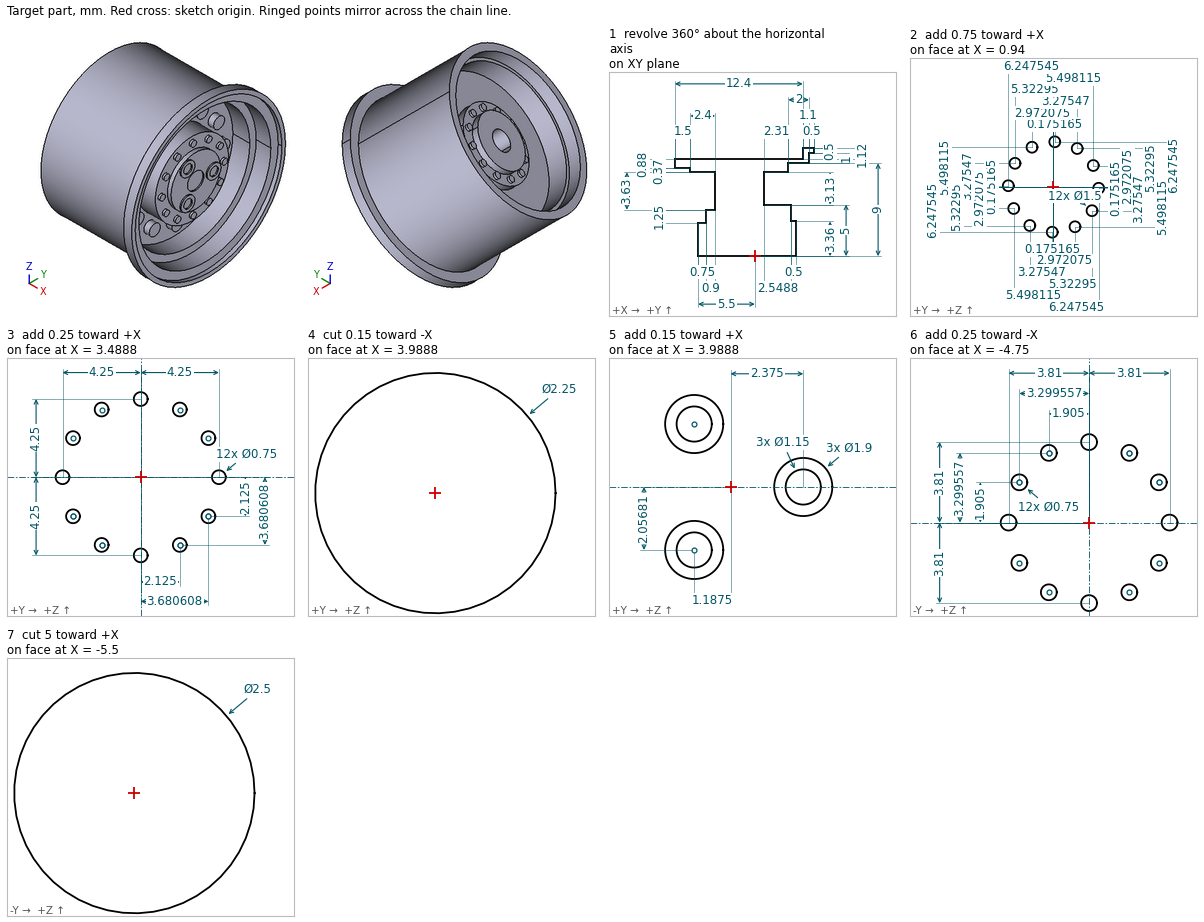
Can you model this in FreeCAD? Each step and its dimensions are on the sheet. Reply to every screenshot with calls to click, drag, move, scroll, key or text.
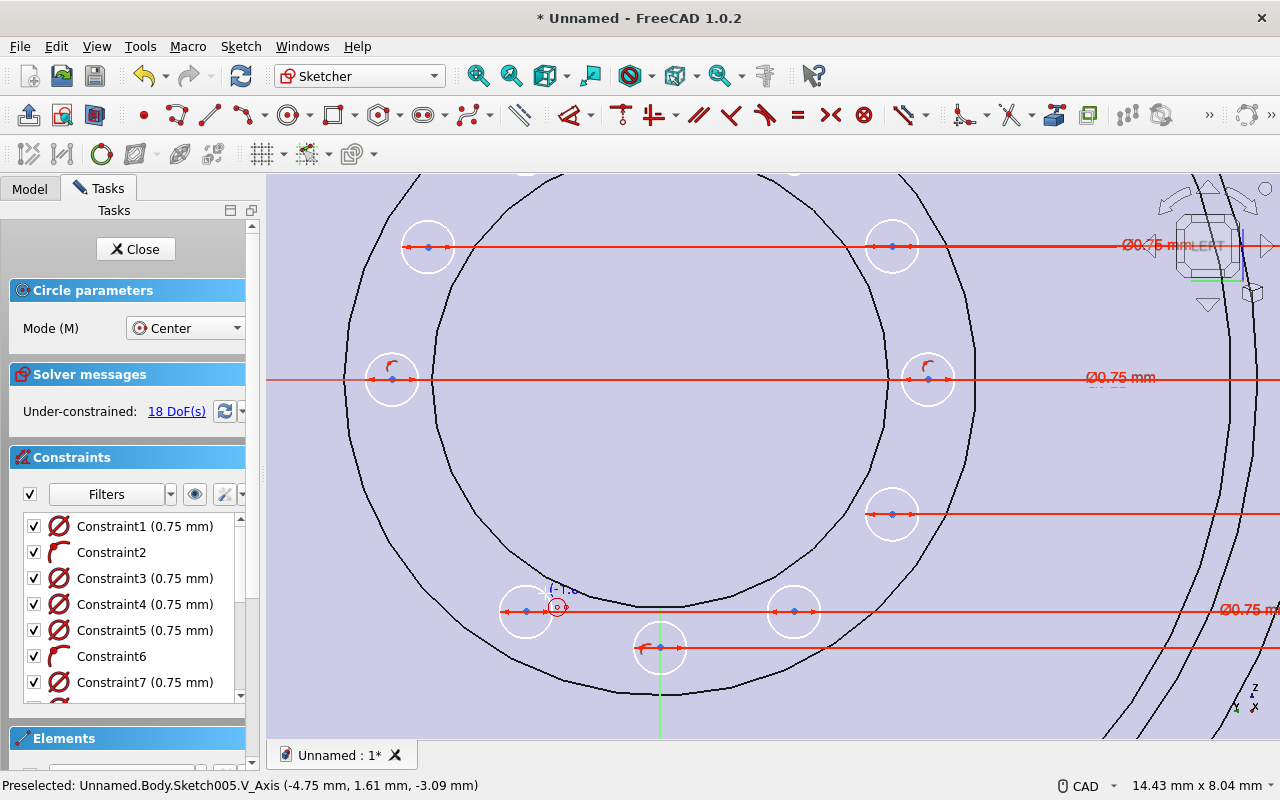
click(428, 513)
move(447, 495)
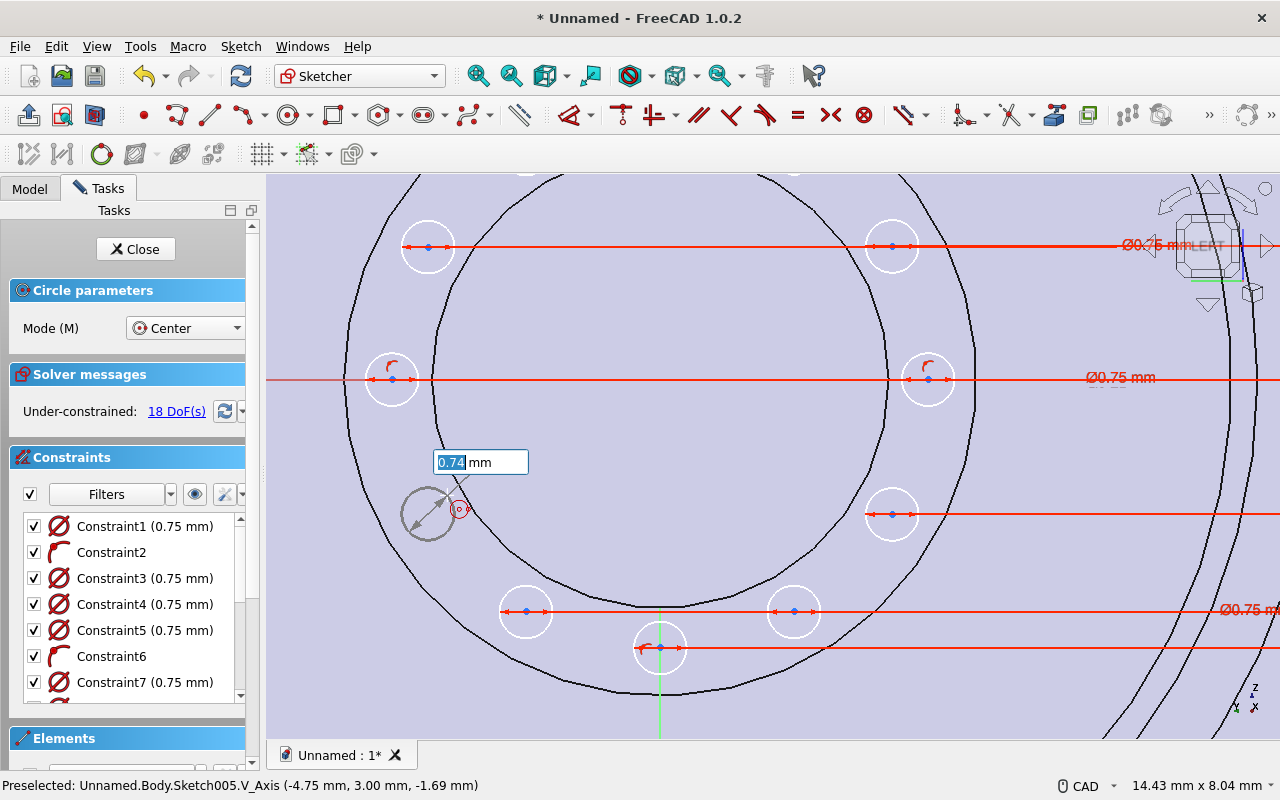
text(0.75)
key(Return)
key(Escape)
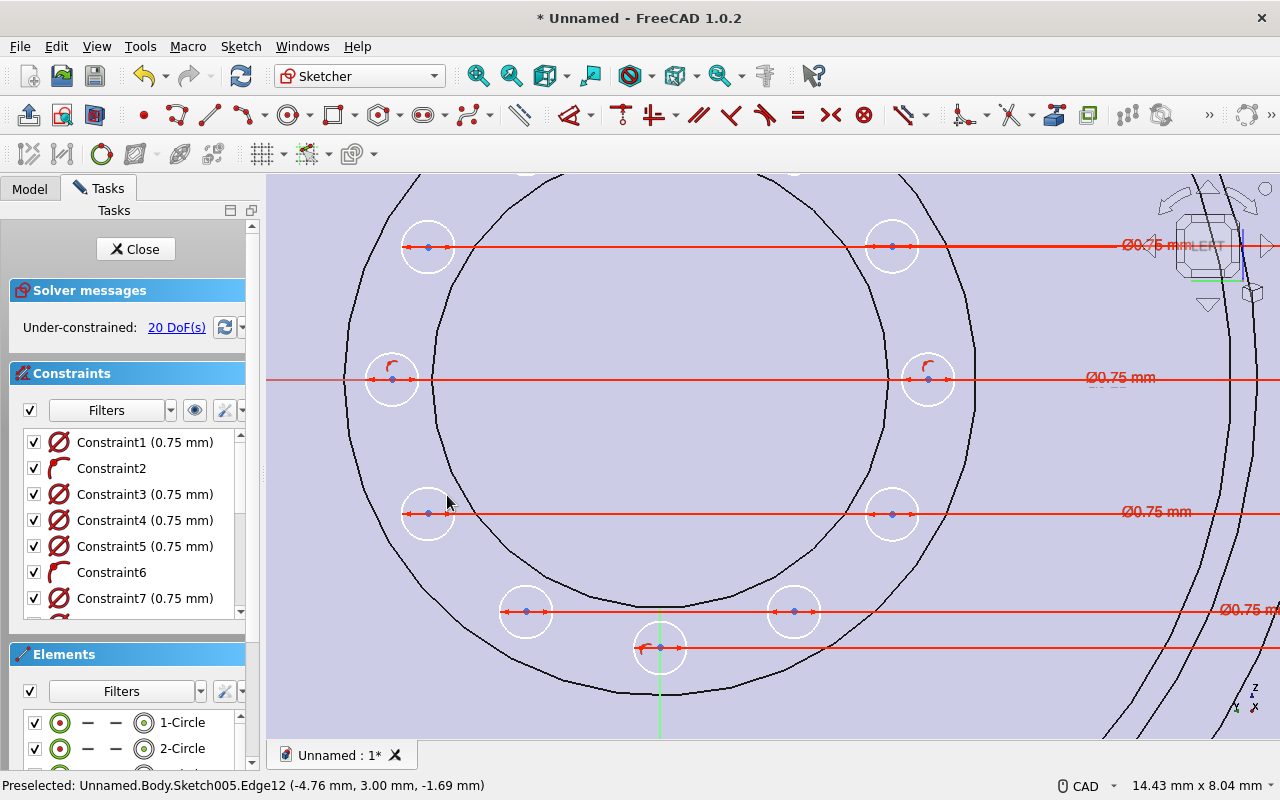
scroll(794, 613, down, 2)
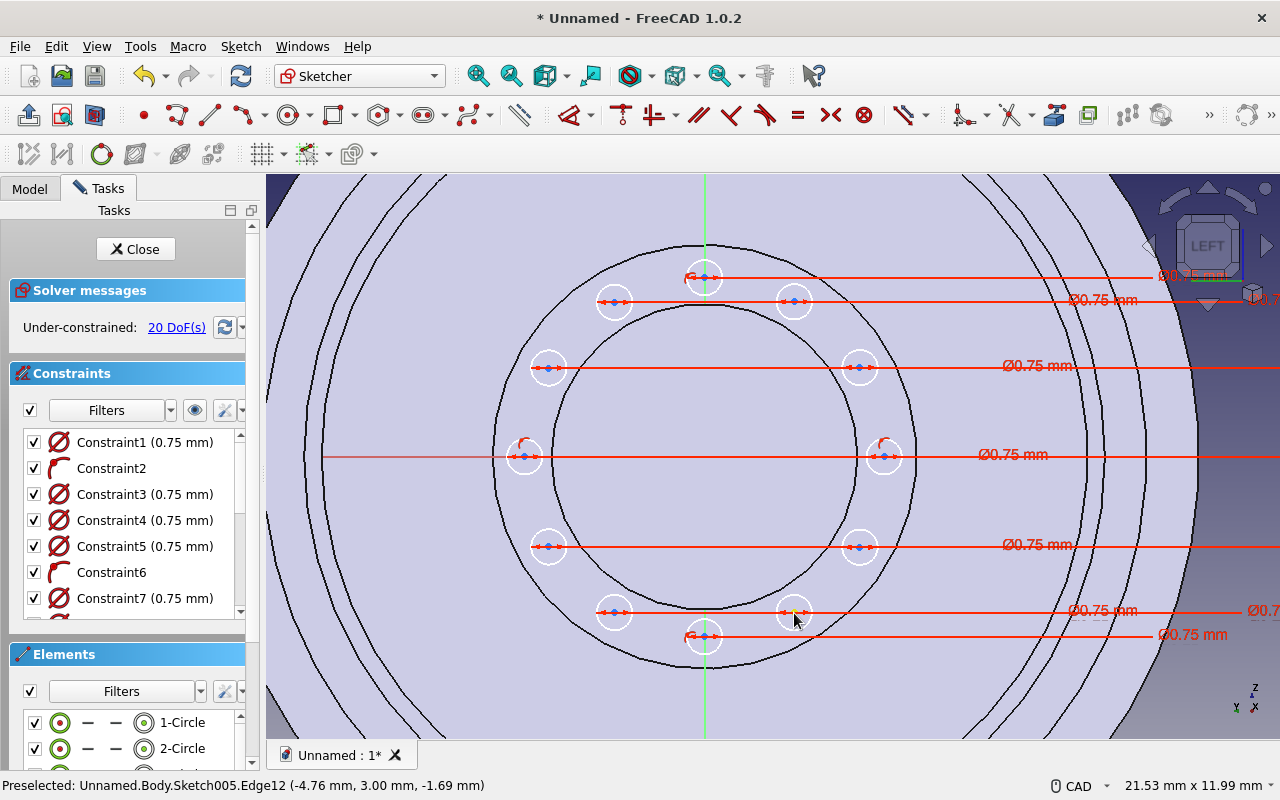
click(615, 302)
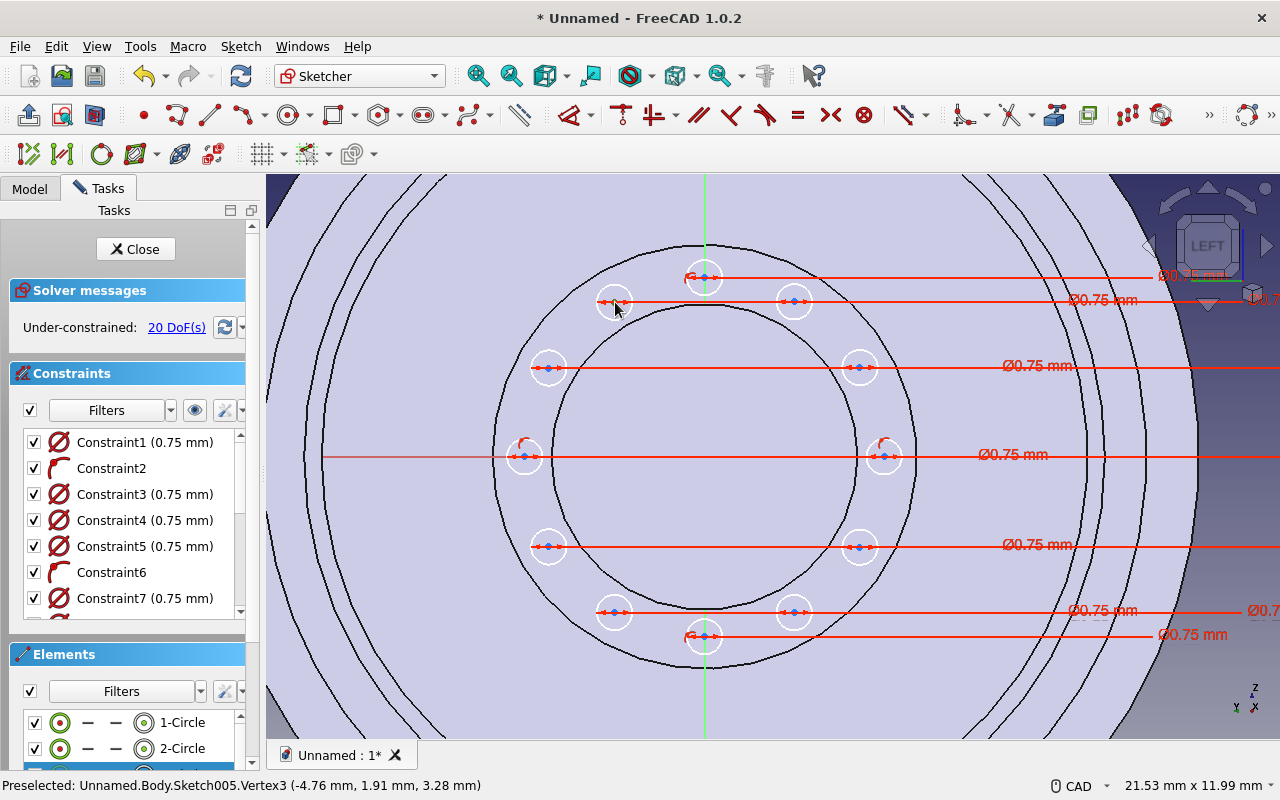
click(794, 302)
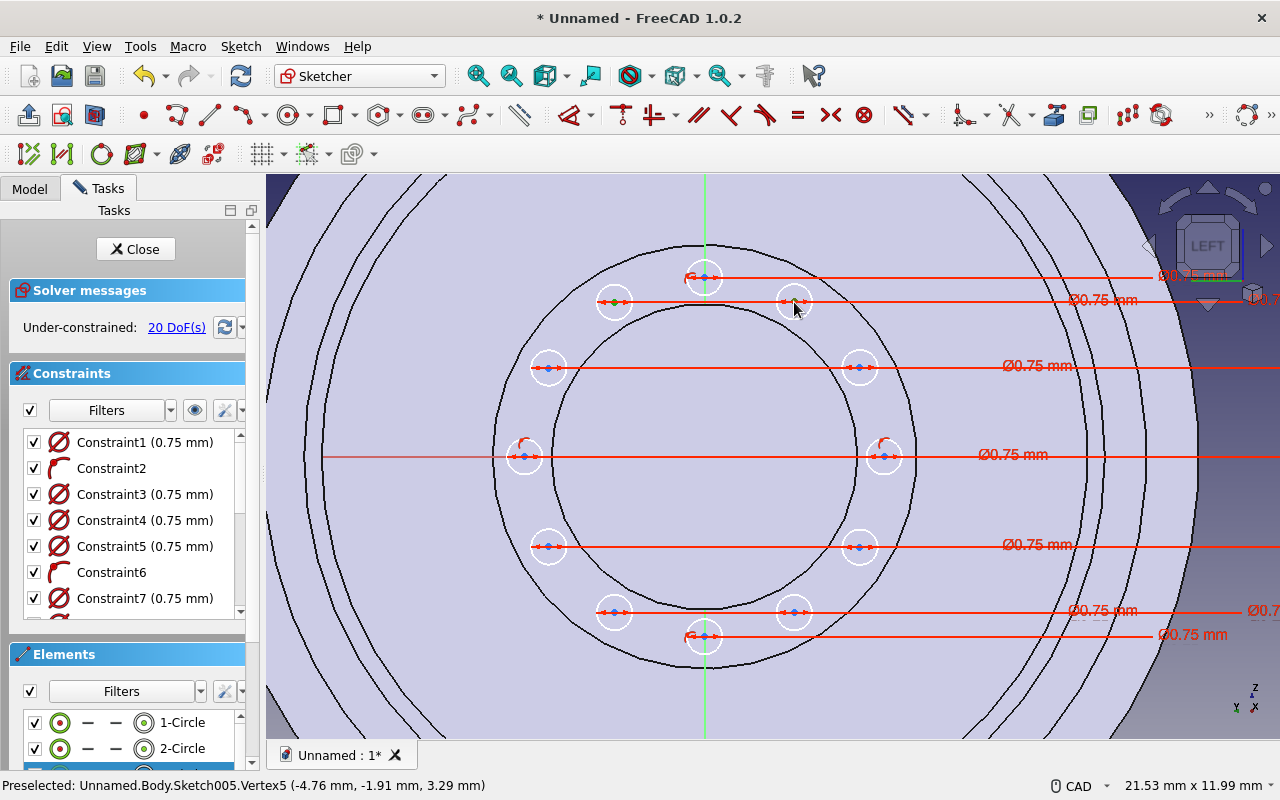
click(705, 566)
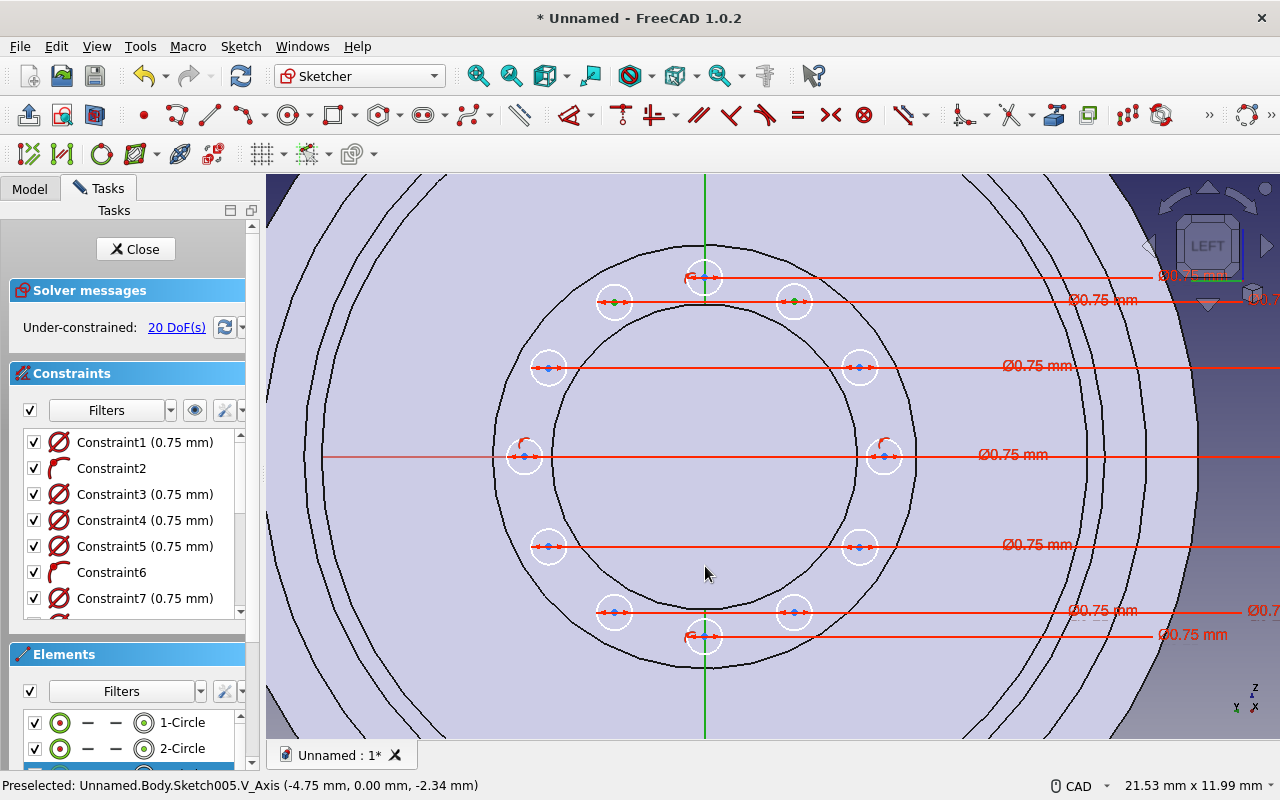
click(831, 116)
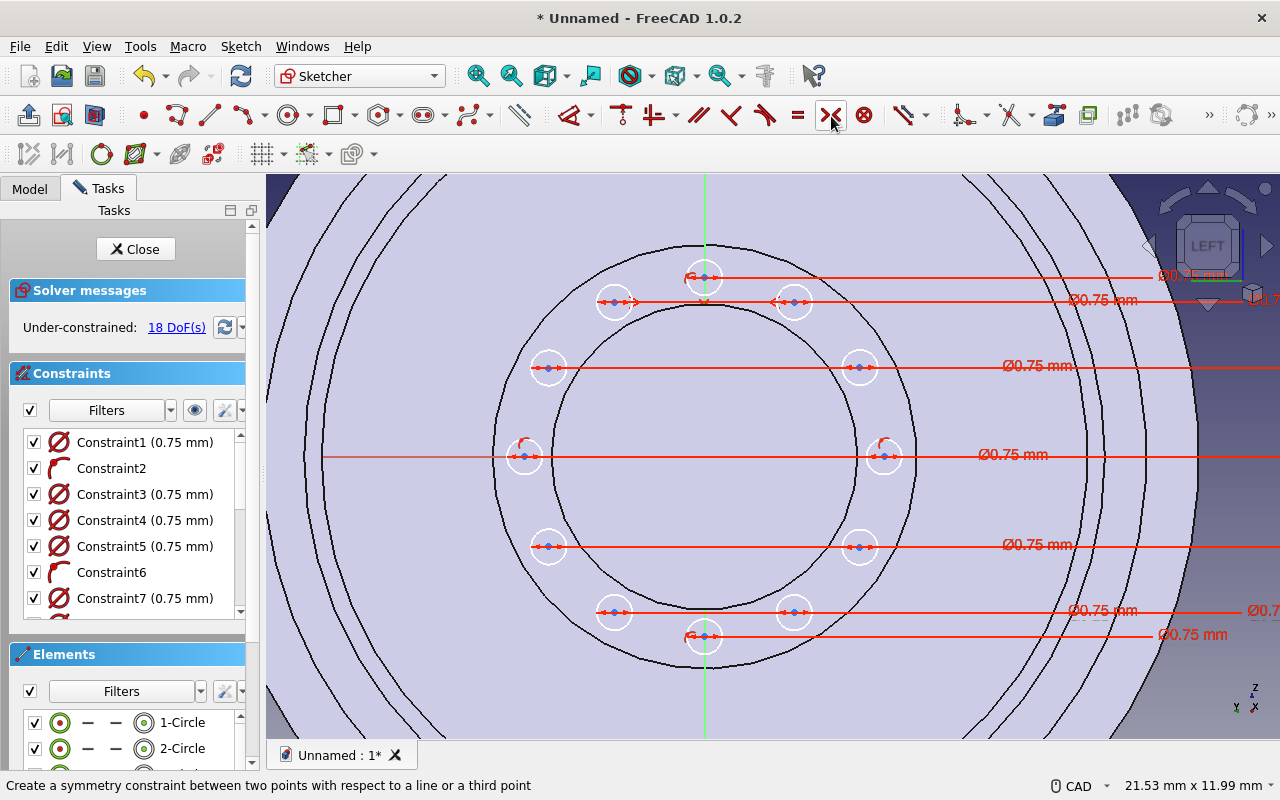
click(549, 368)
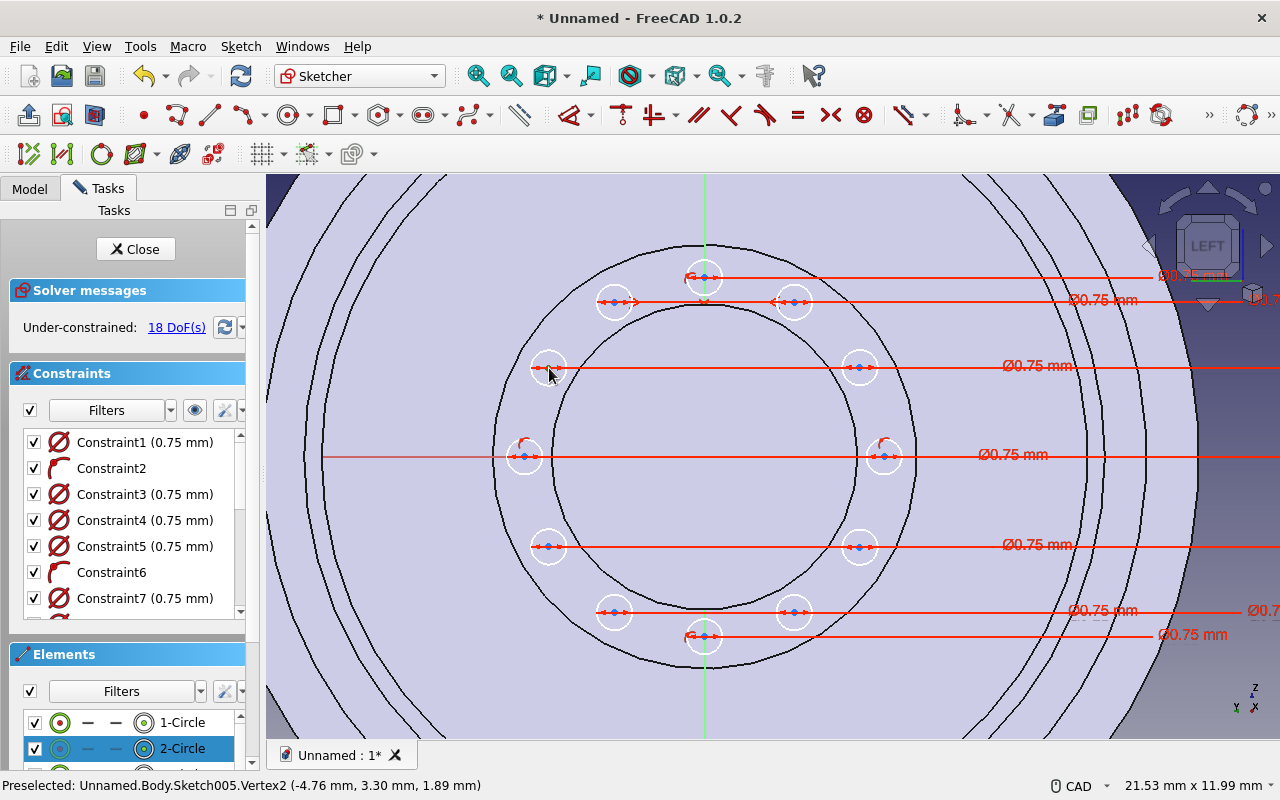
click(860, 368)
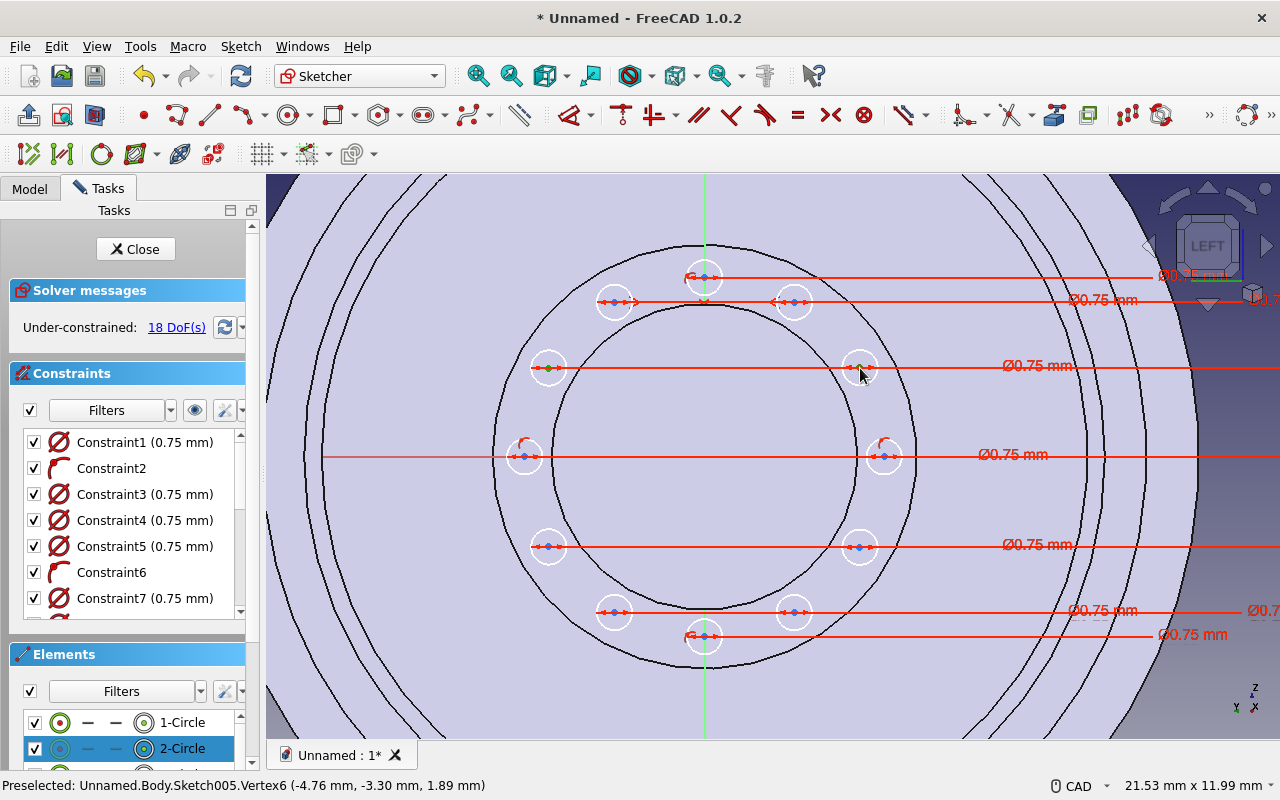
click(705, 566)